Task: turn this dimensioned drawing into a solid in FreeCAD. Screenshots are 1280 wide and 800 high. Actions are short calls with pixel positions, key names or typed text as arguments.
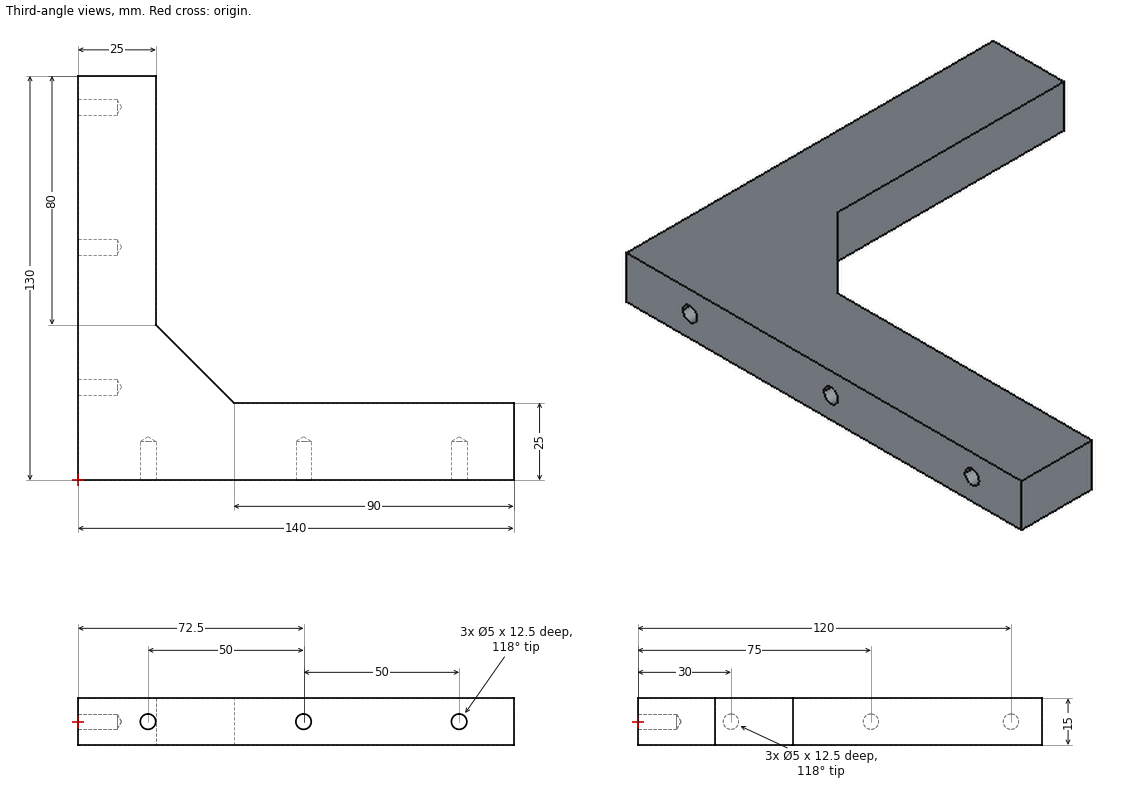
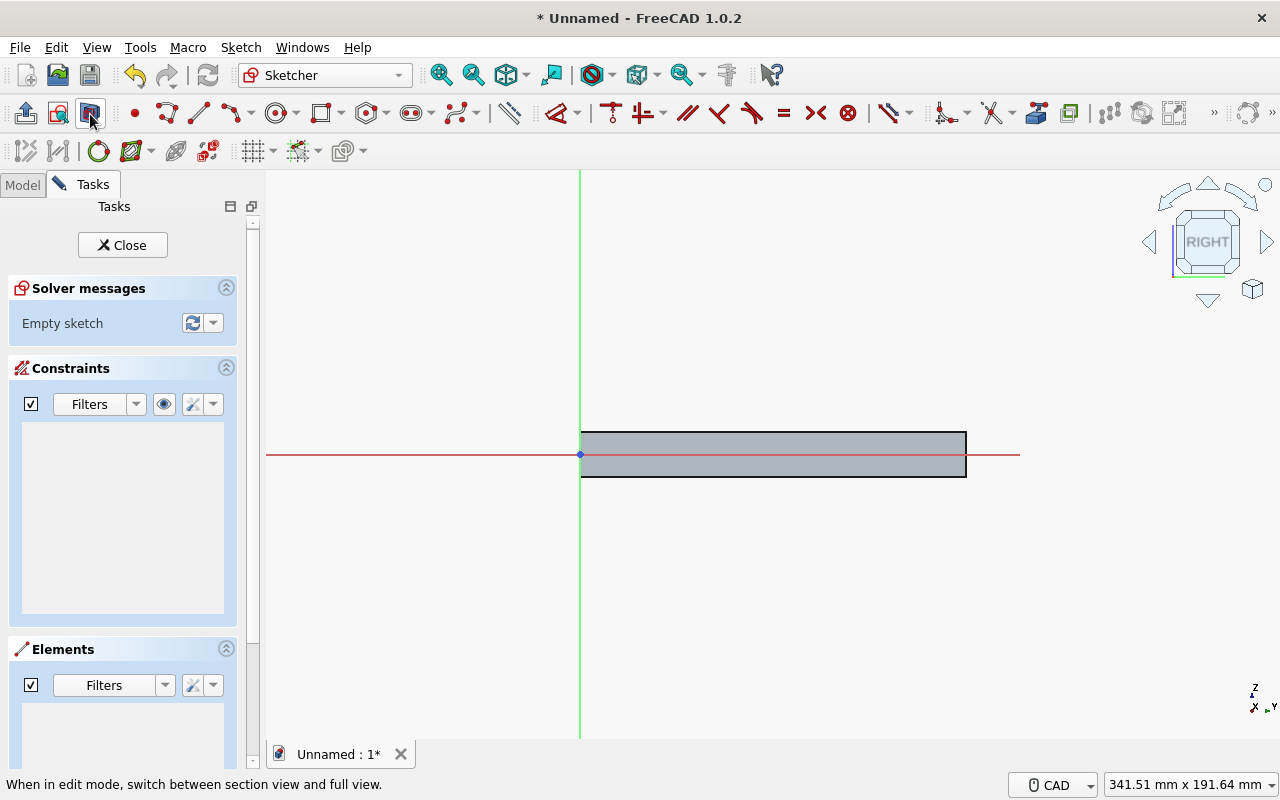
scroll(879, 455, up, 2)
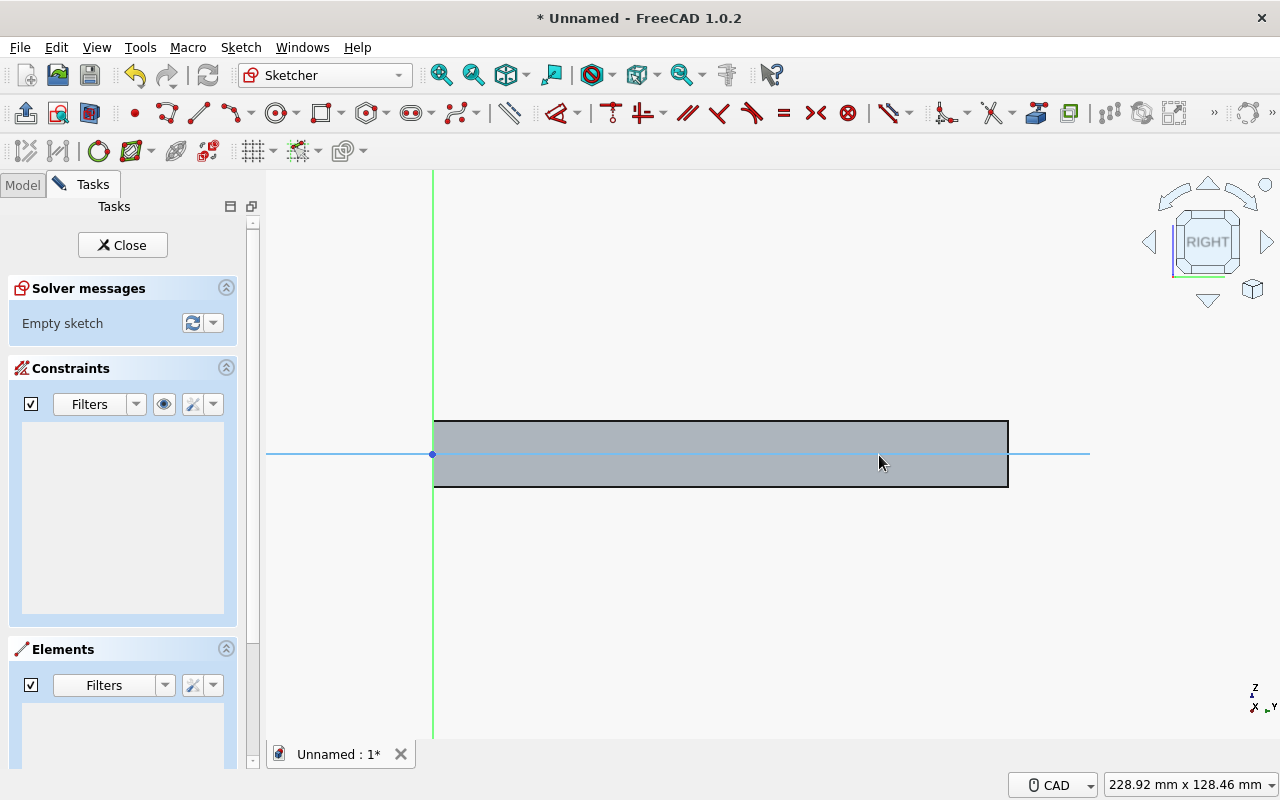
click(276, 114)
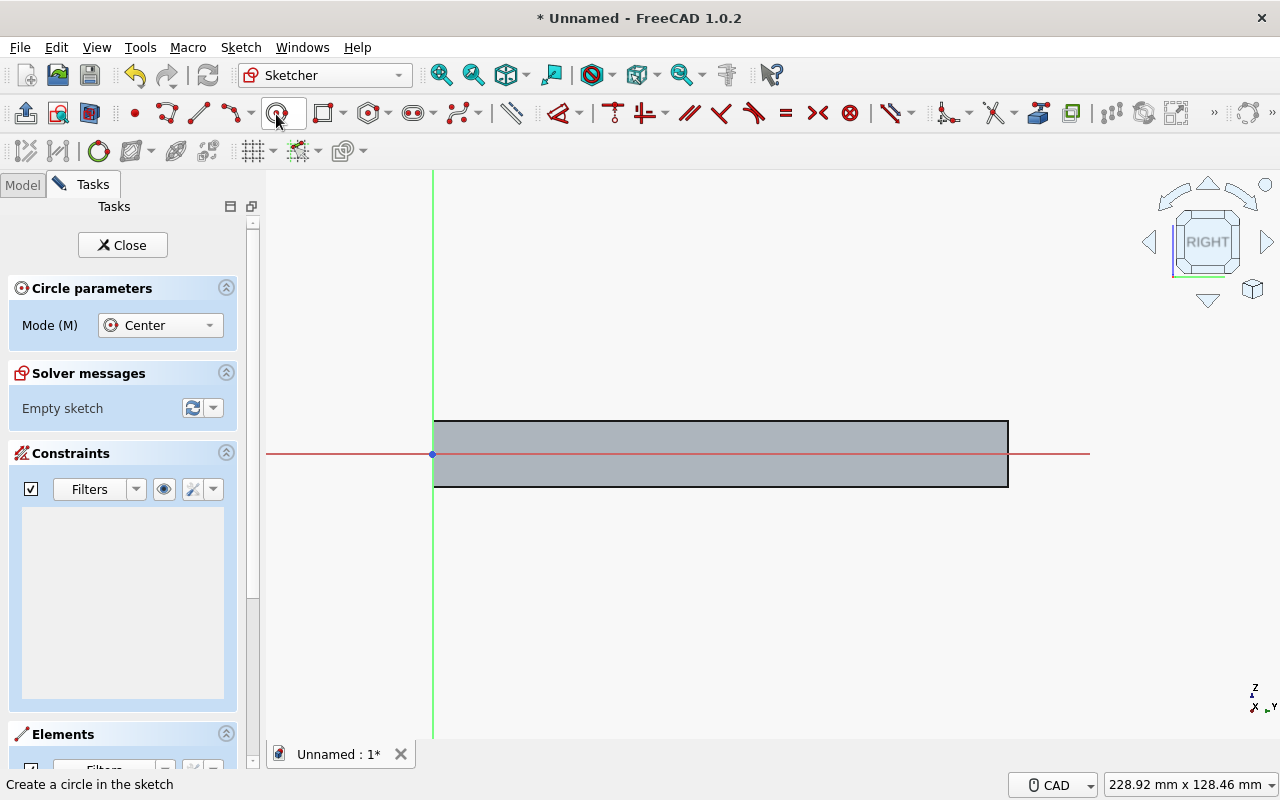
scroll(566, 454, up, 4)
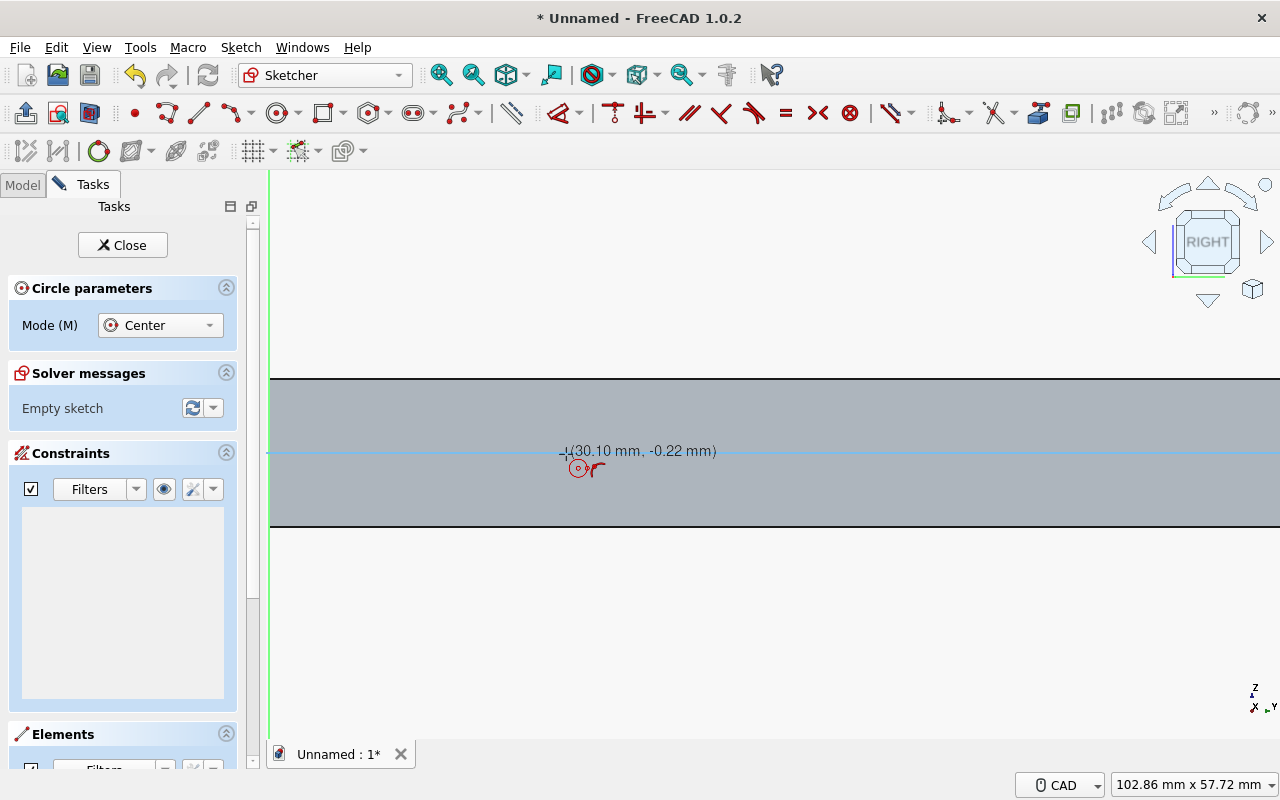
click(565, 453)
click(582, 436)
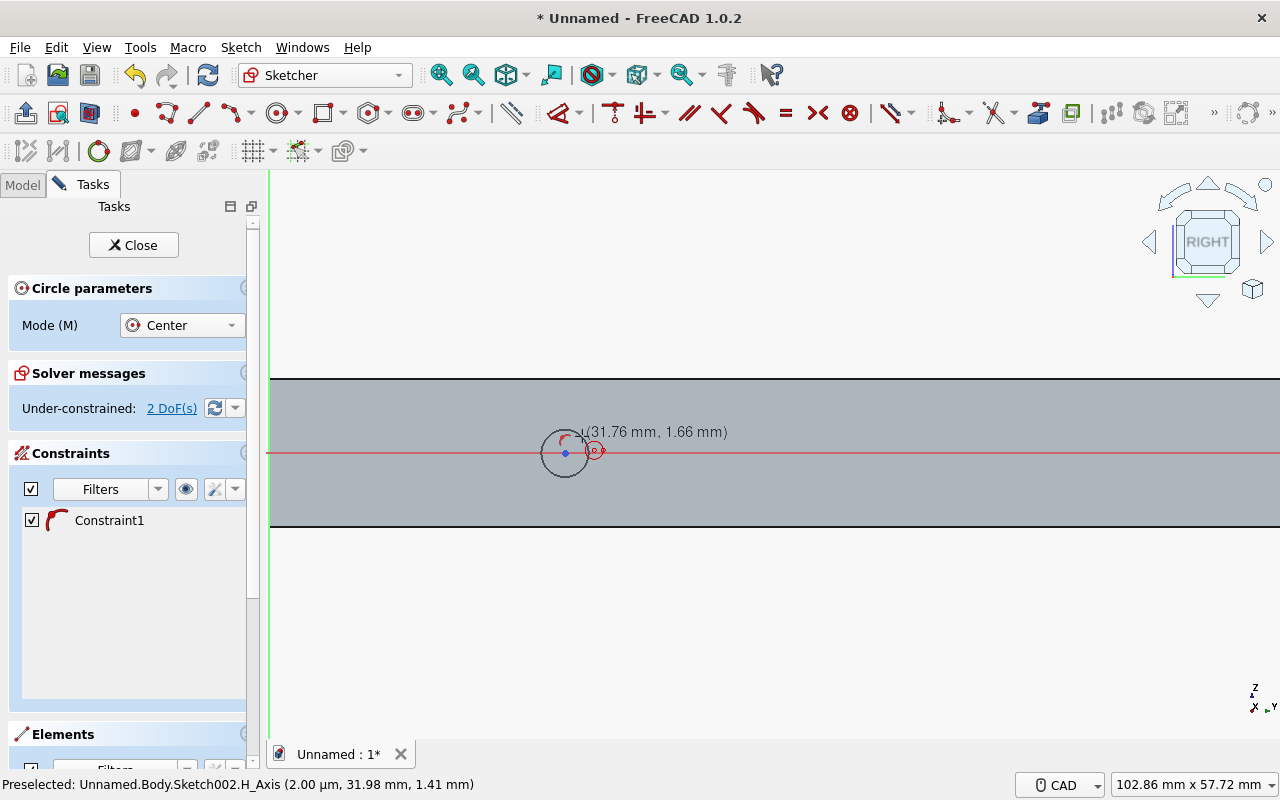
click(1008, 453)
click(1026, 436)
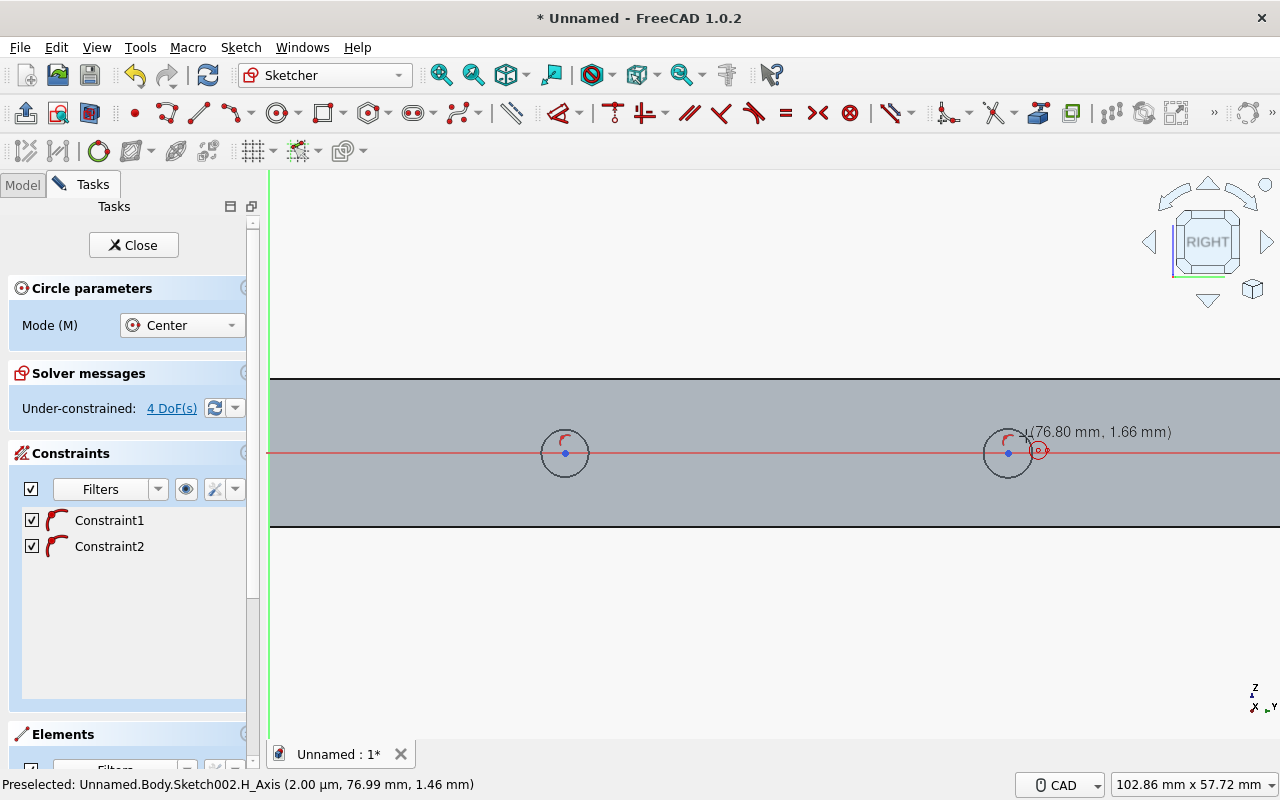
scroll(567, 455, down, 4)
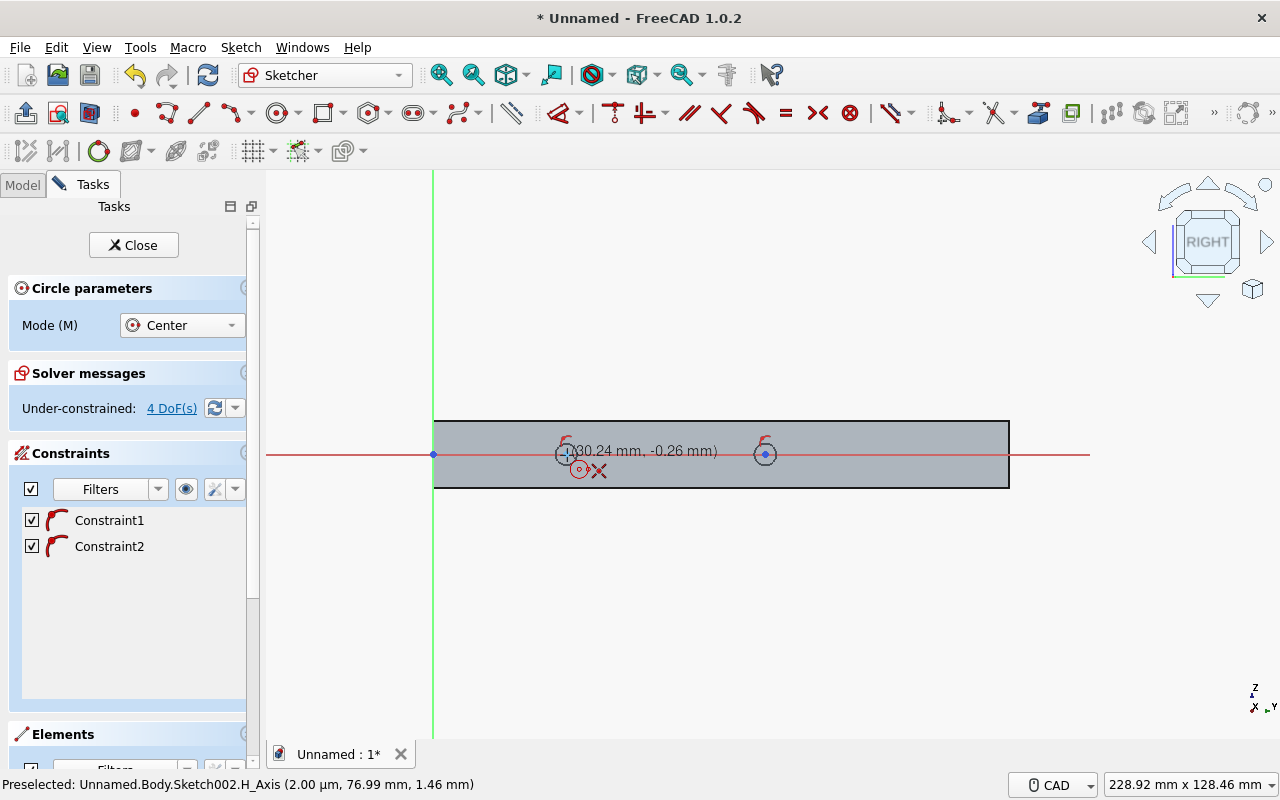
scroll(965, 455, up, 4)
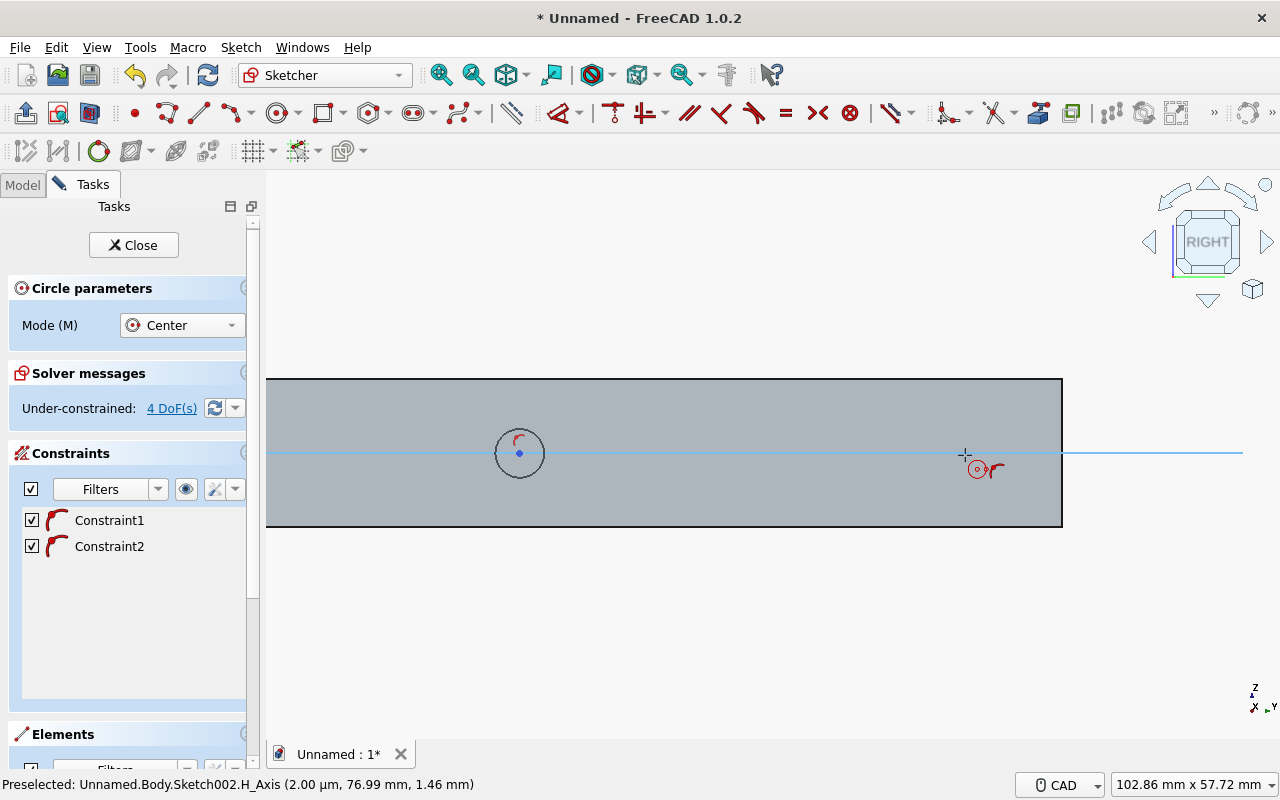
click(964, 453)
click(981, 436)
key(Escape)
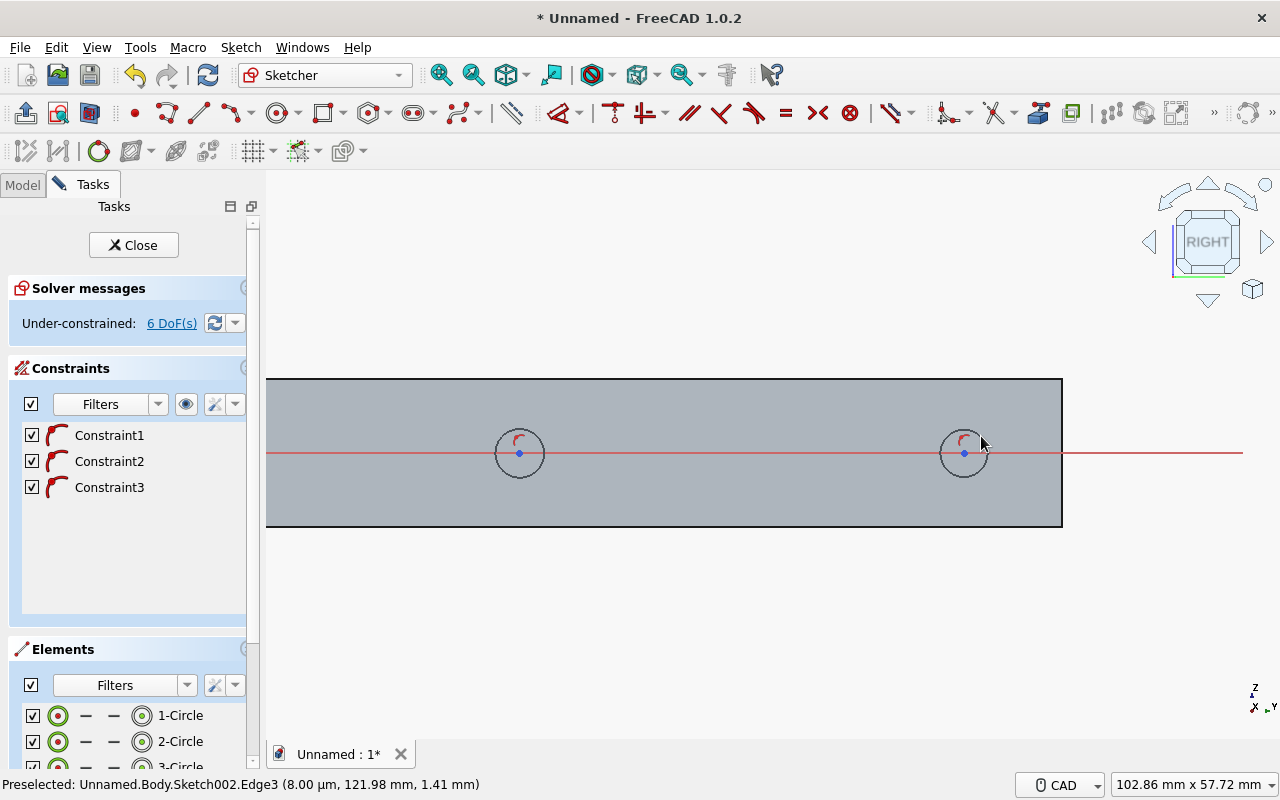
scroll(966, 455, down, 4)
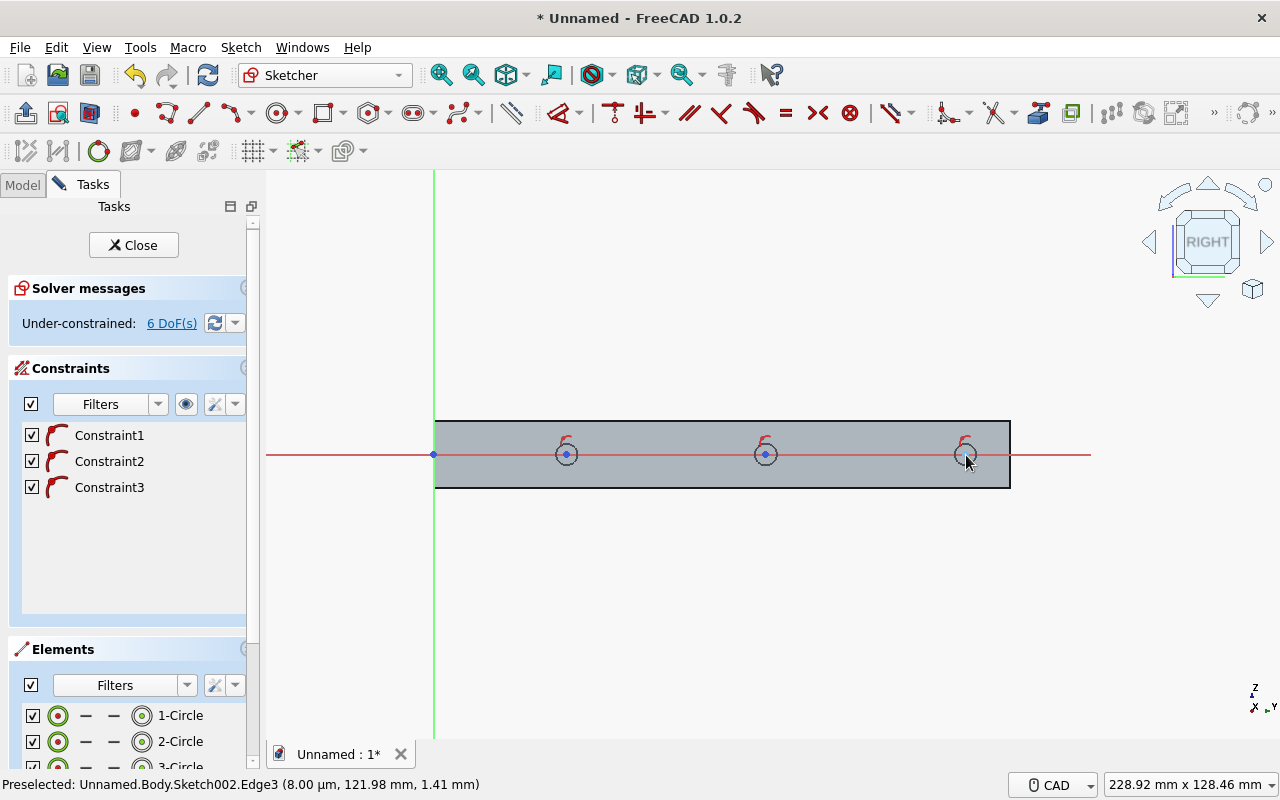
scroll(574, 447, up, 4)